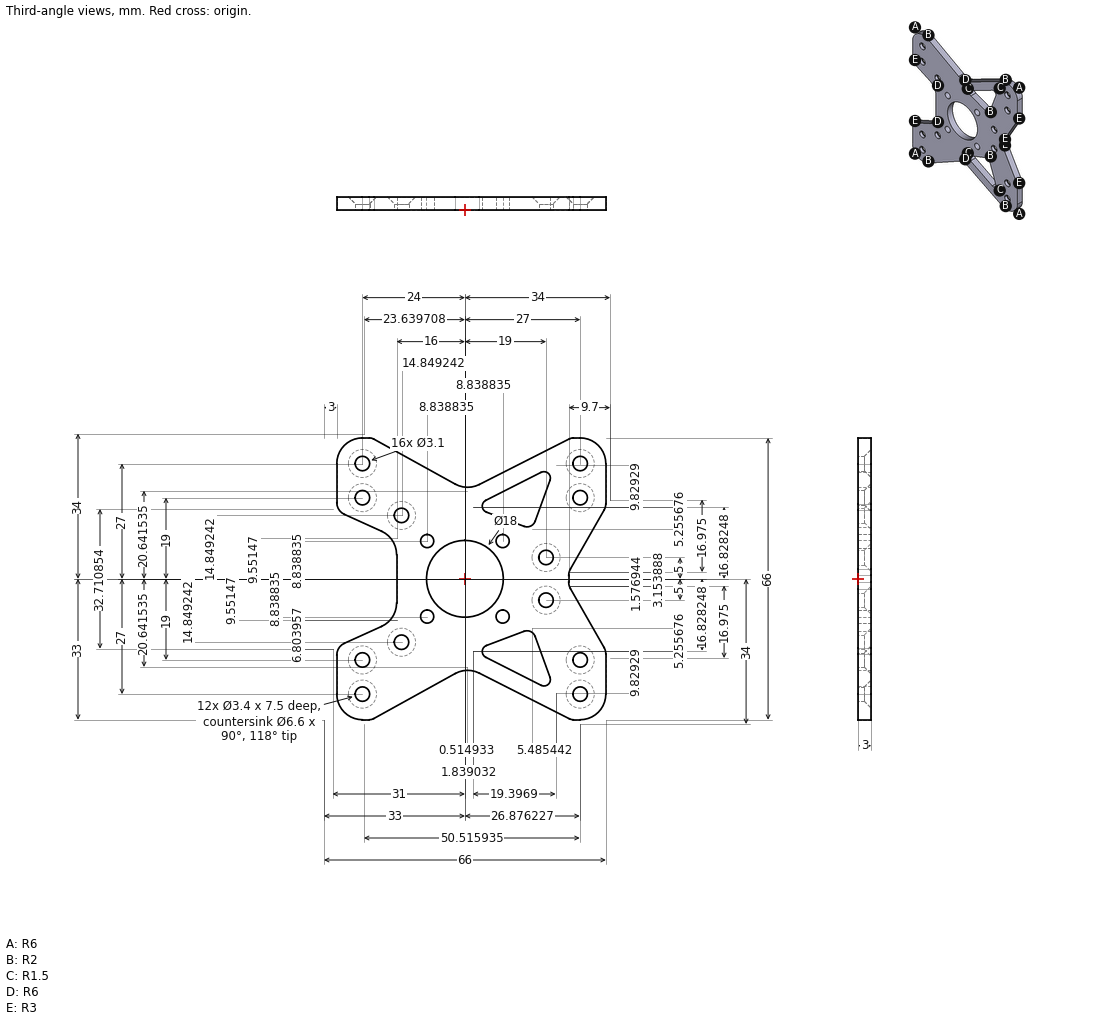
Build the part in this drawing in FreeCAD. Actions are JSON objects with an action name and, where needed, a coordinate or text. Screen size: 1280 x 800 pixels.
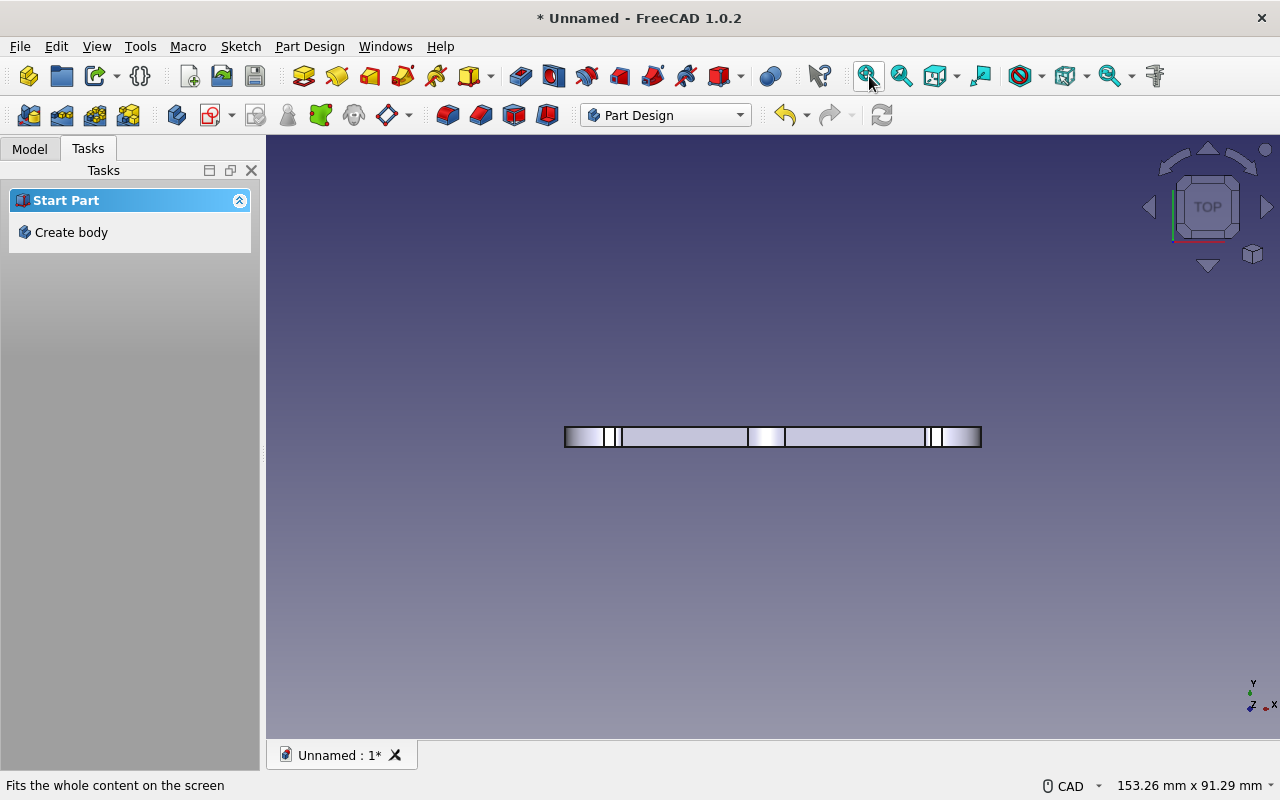
{"action": "key", "text": "0"}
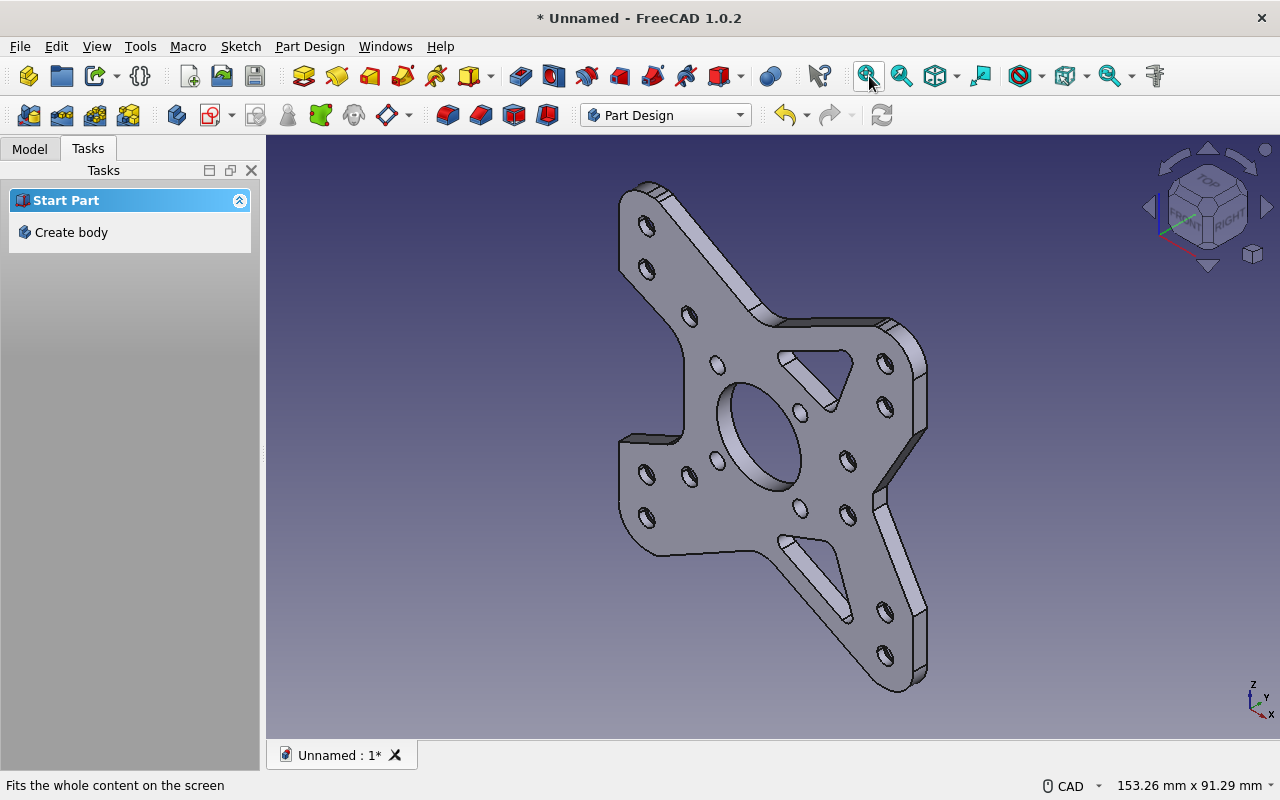
{"action": "scroll", "coordinate": [626, 437], "scroll_direction": "up", "scroll_amount": 4}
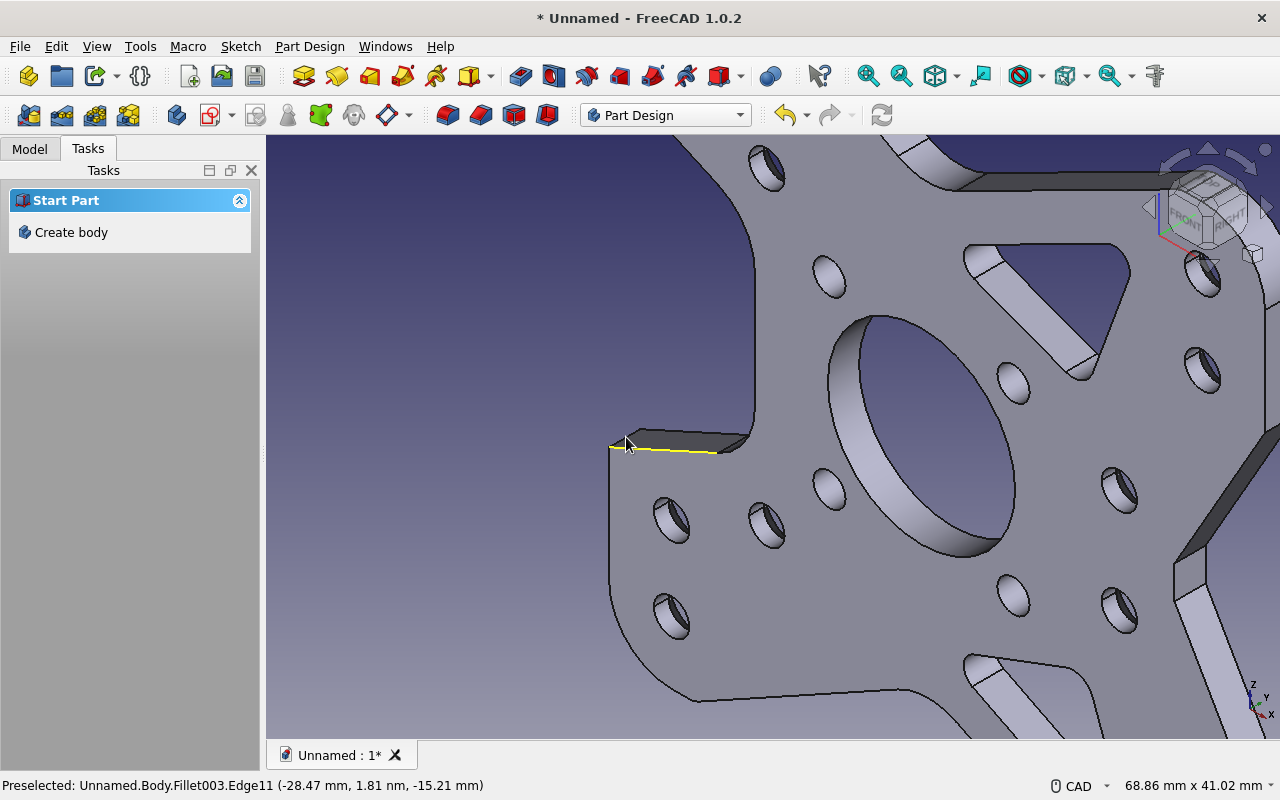
{"action": "left_click", "coordinate": [869, 76]}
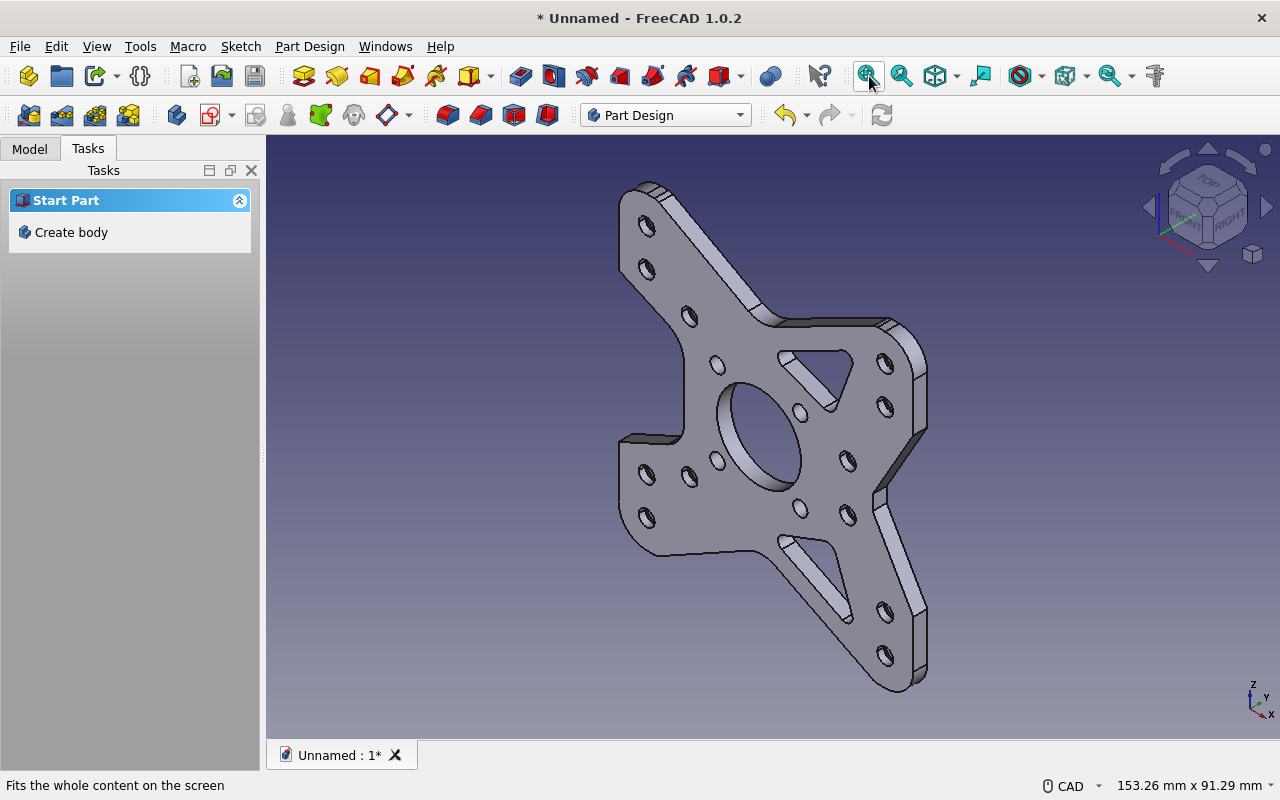
{"action": "key", "text": "1"}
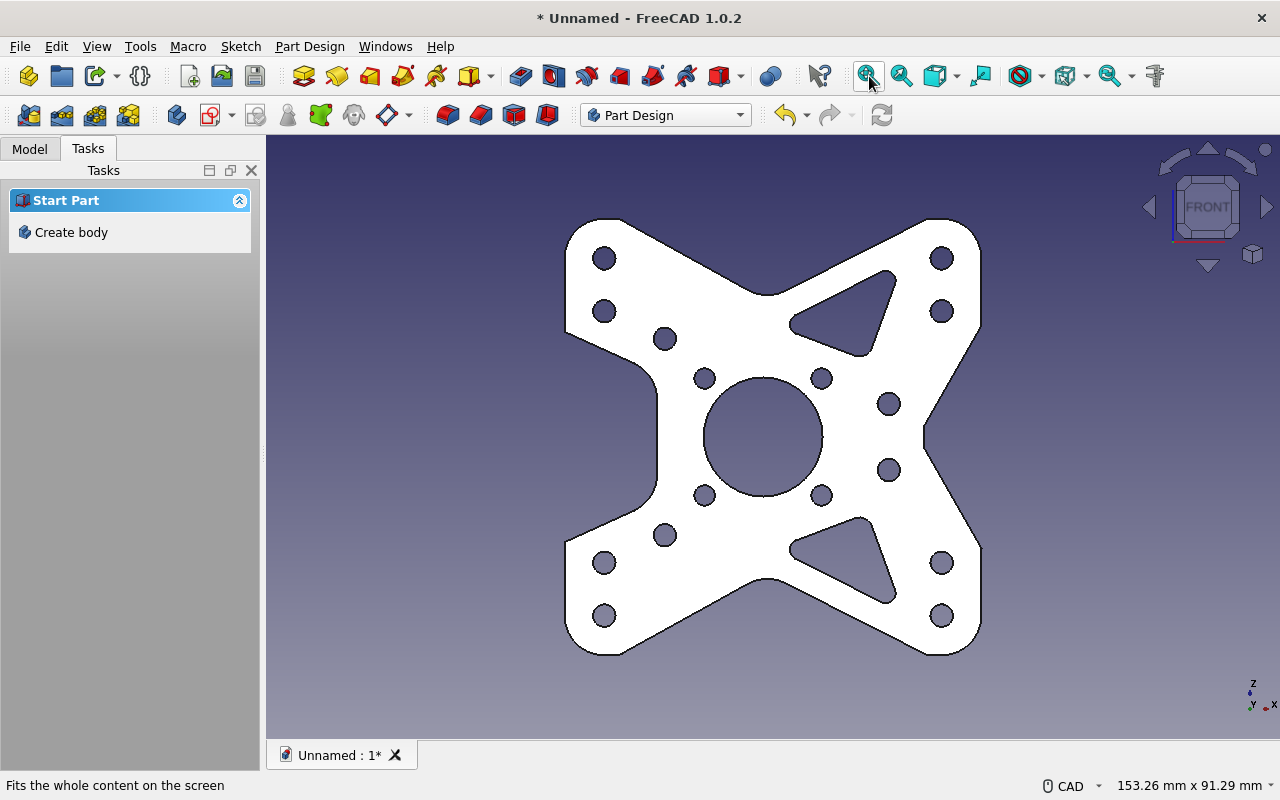
{"action": "scroll", "coordinate": [565, 541], "scroll_direction": "up", "scroll_amount": 4}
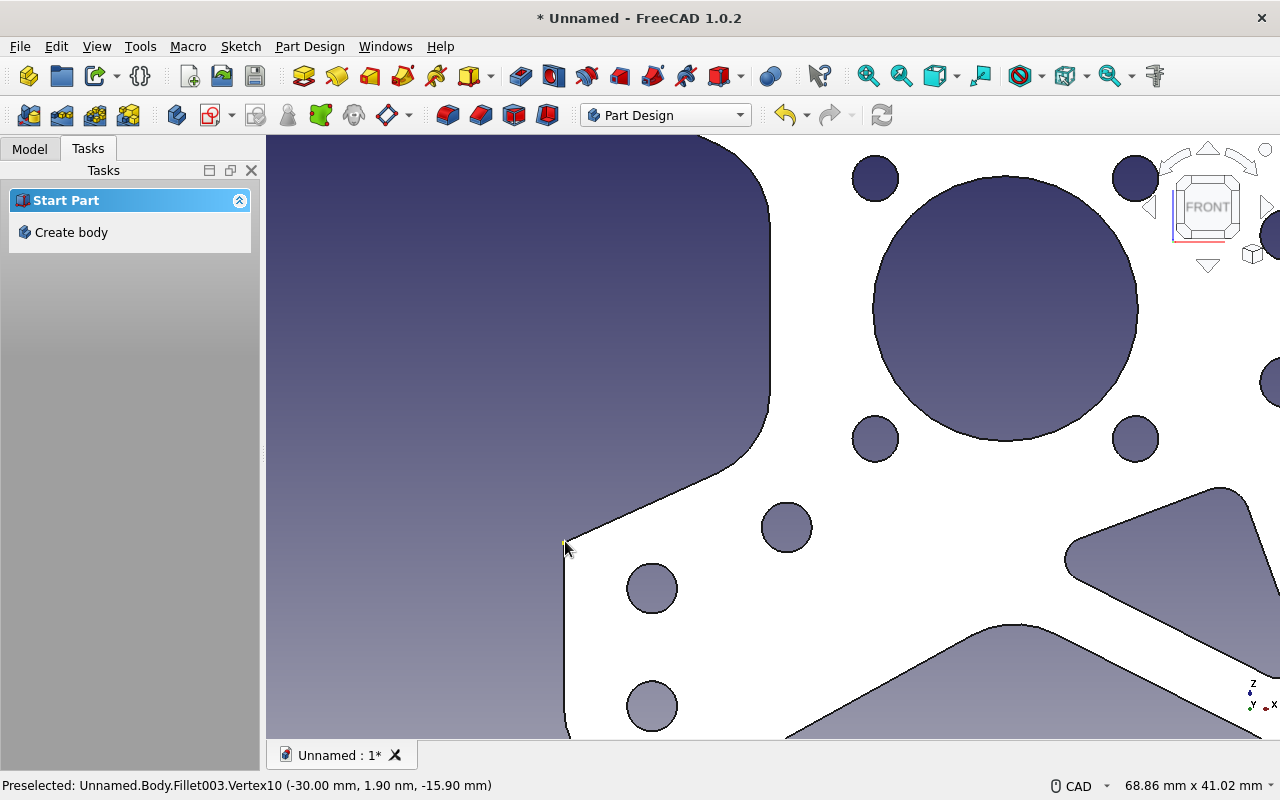
{"action": "key", "text": "v f"}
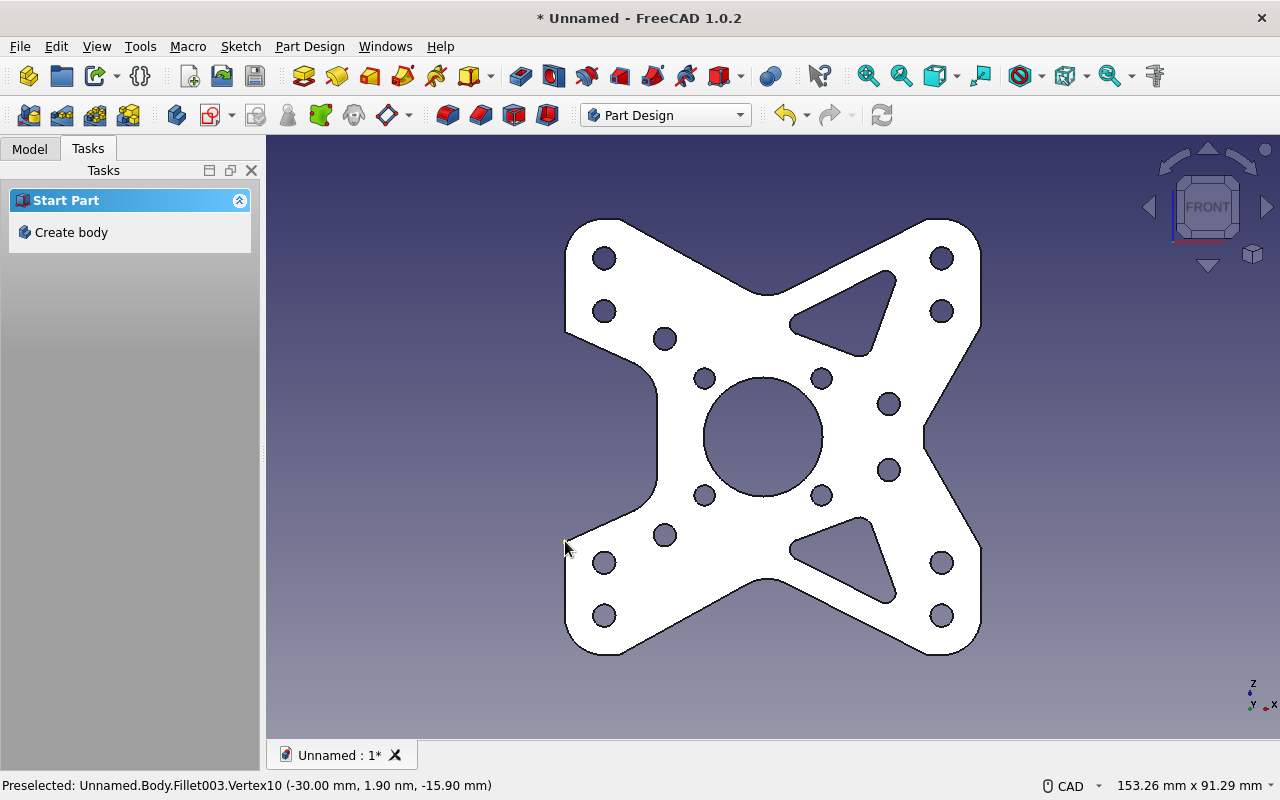
{"action": "key", "text": "3"}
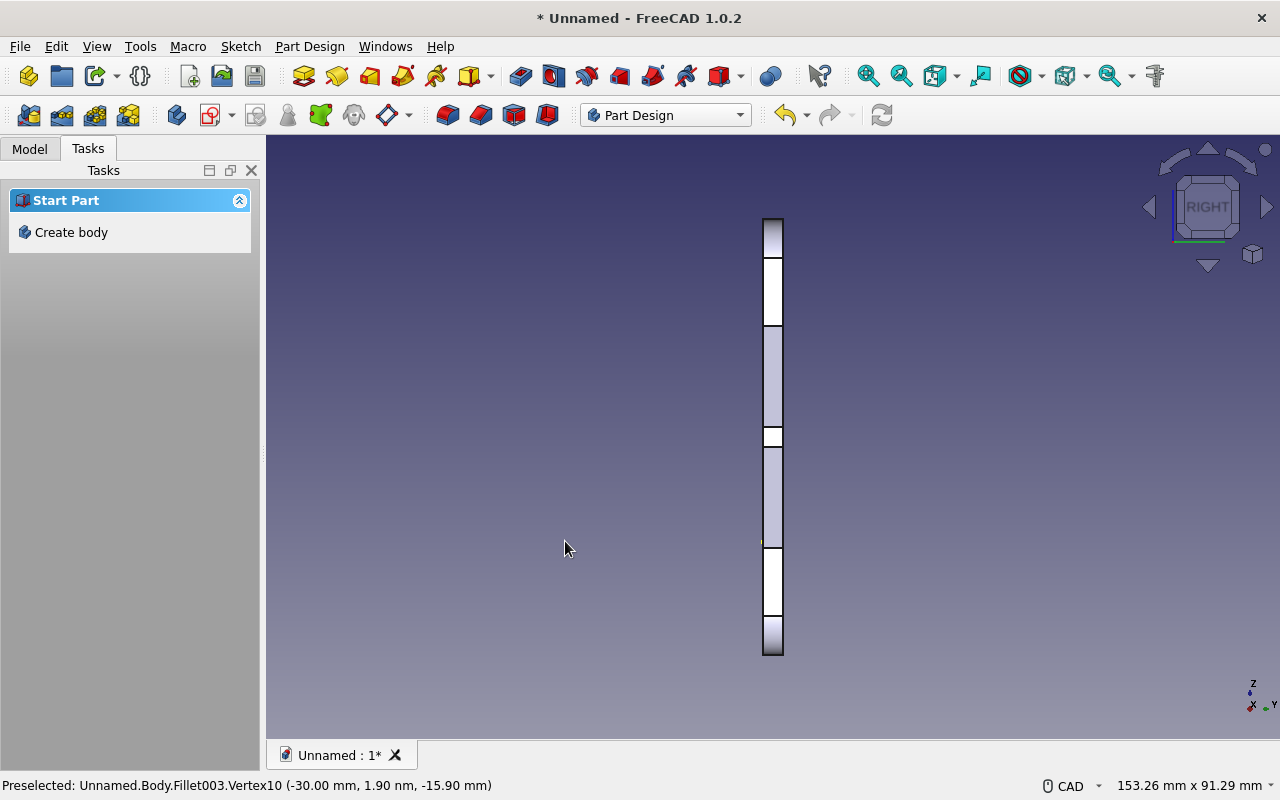
{"action": "left_click", "coordinate": [773, 325]}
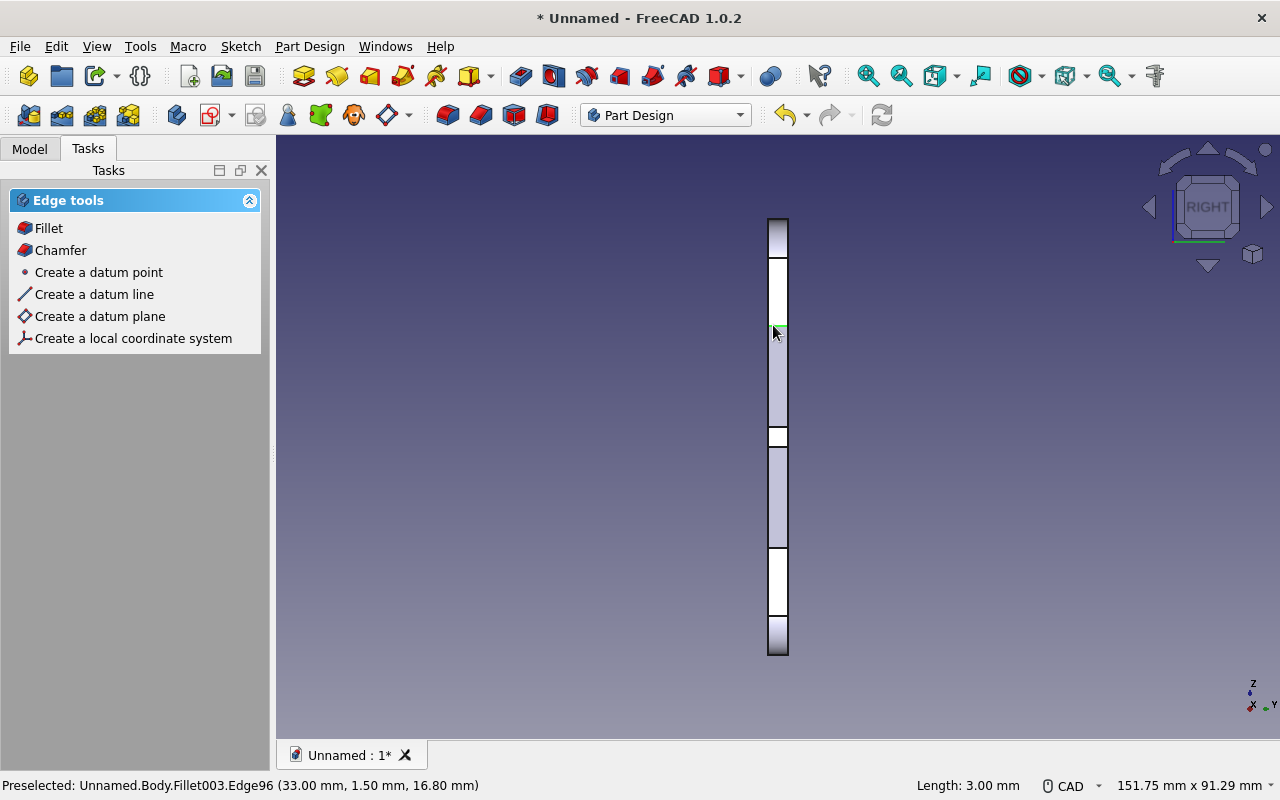
{"action": "left_click", "coordinate": [778, 547], "text": "ctrl"}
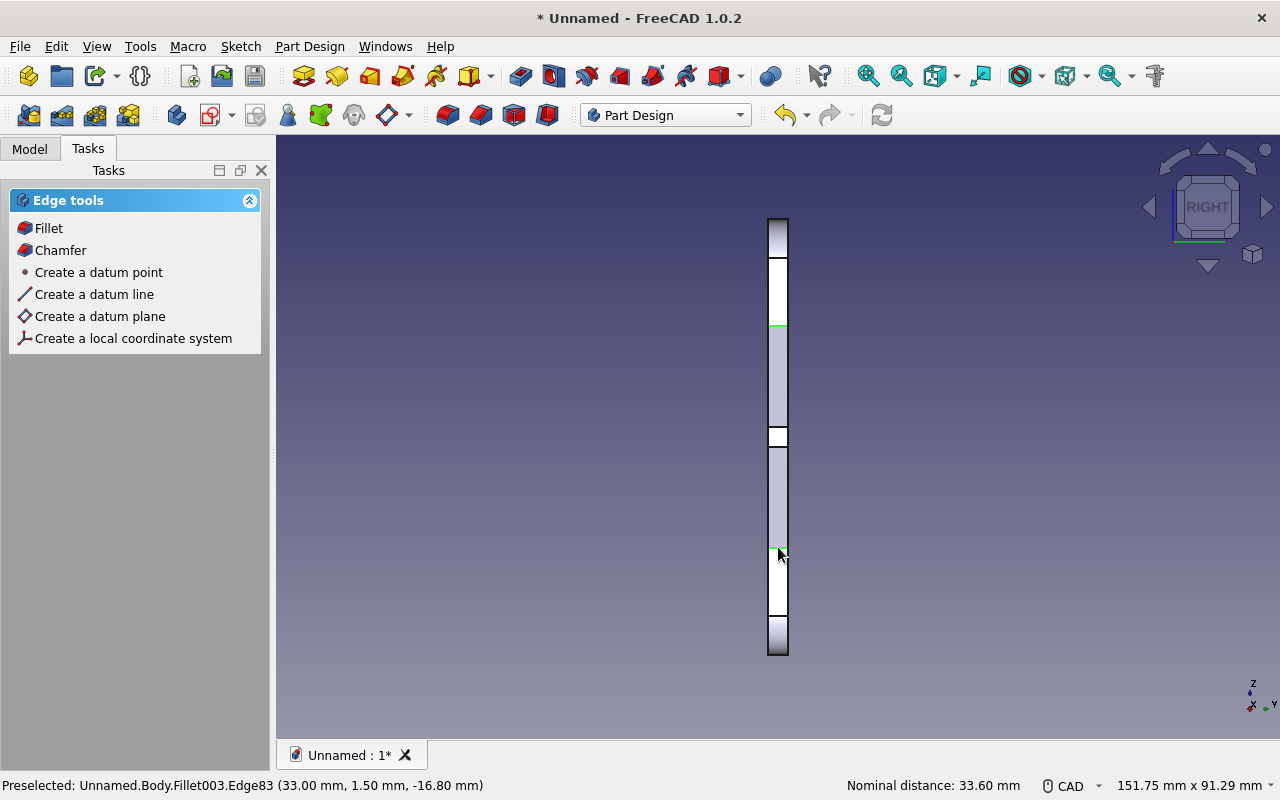
{"action": "scroll", "coordinate": [778, 541], "scroll_direction": "up", "scroll_amount": 4}